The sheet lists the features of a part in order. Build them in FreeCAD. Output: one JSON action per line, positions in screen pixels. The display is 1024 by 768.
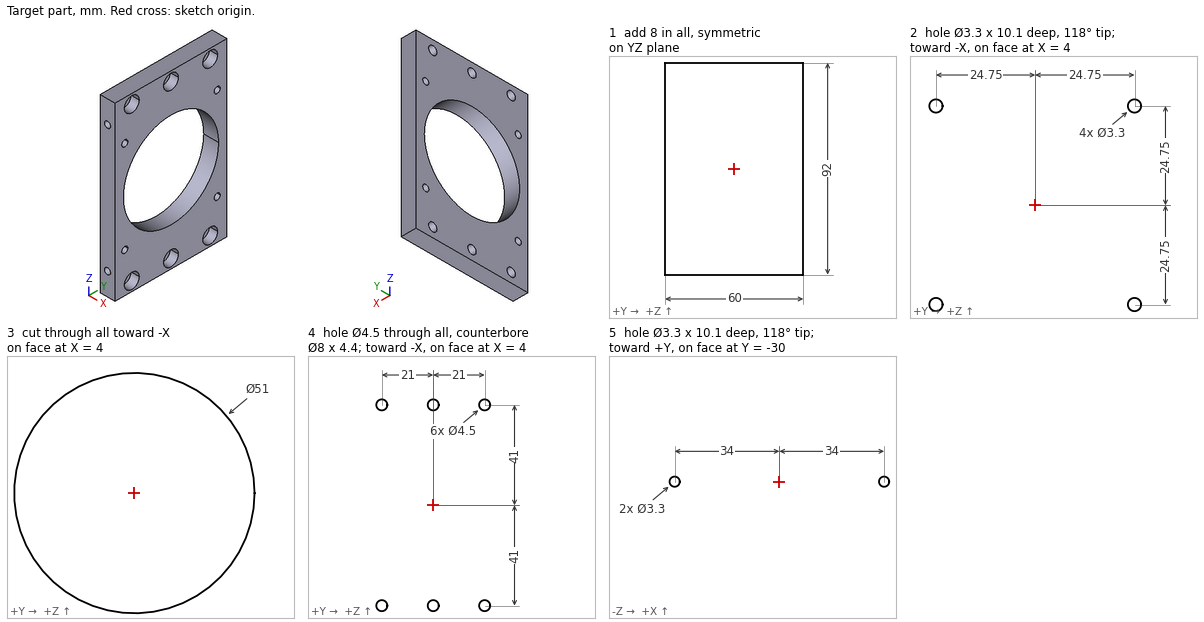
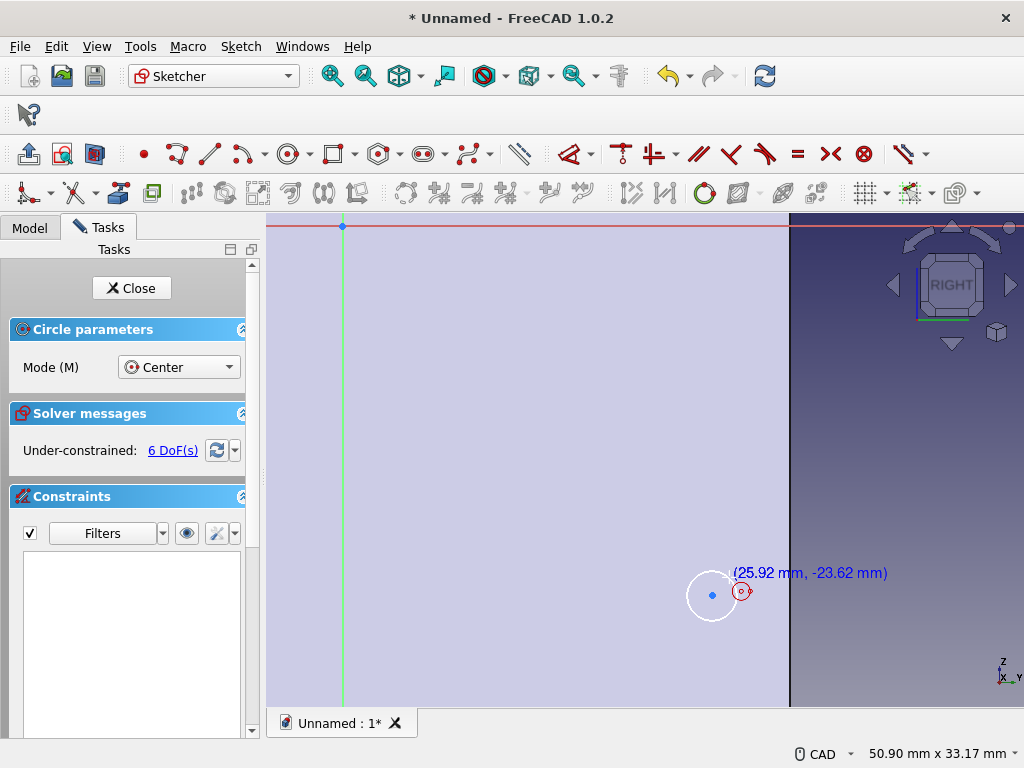
{"action": "scroll", "coordinate": [712, 596], "scroll_direction": "down", "scroll_amount": 5}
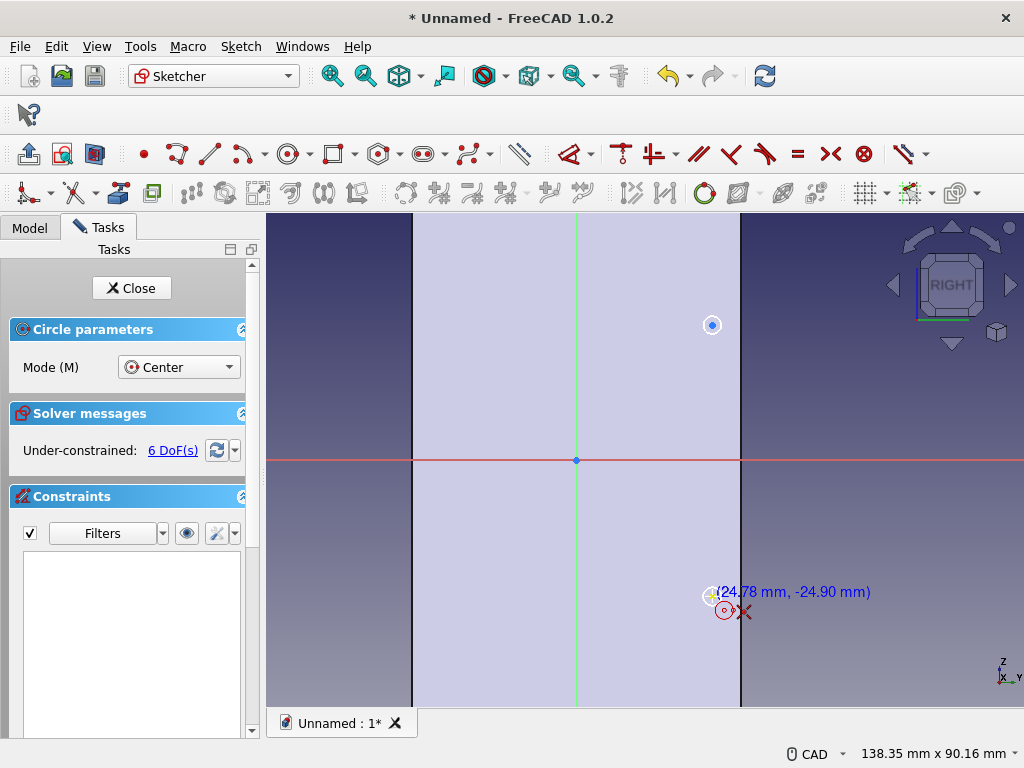
{"action": "scroll", "coordinate": [441, 325], "scroll_direction": "up", "scroll_amount": 5}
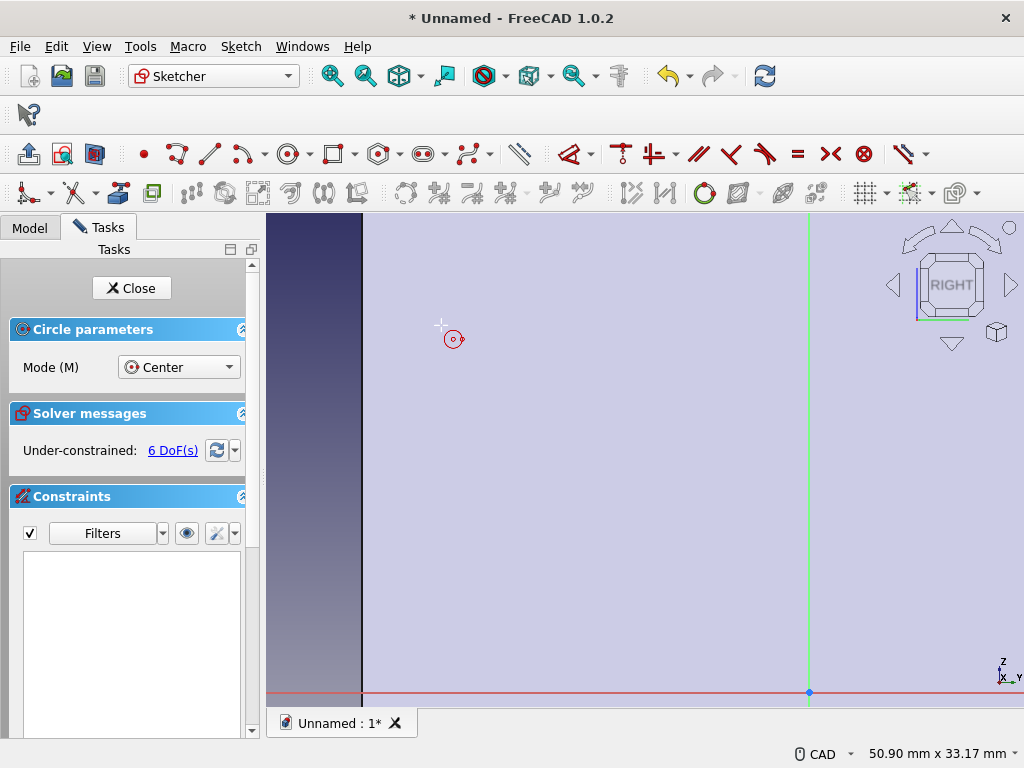
{"action": "left_click", "coordinate": [441, 324]}
{"action": "left_click", "coordinate": [458, 307]}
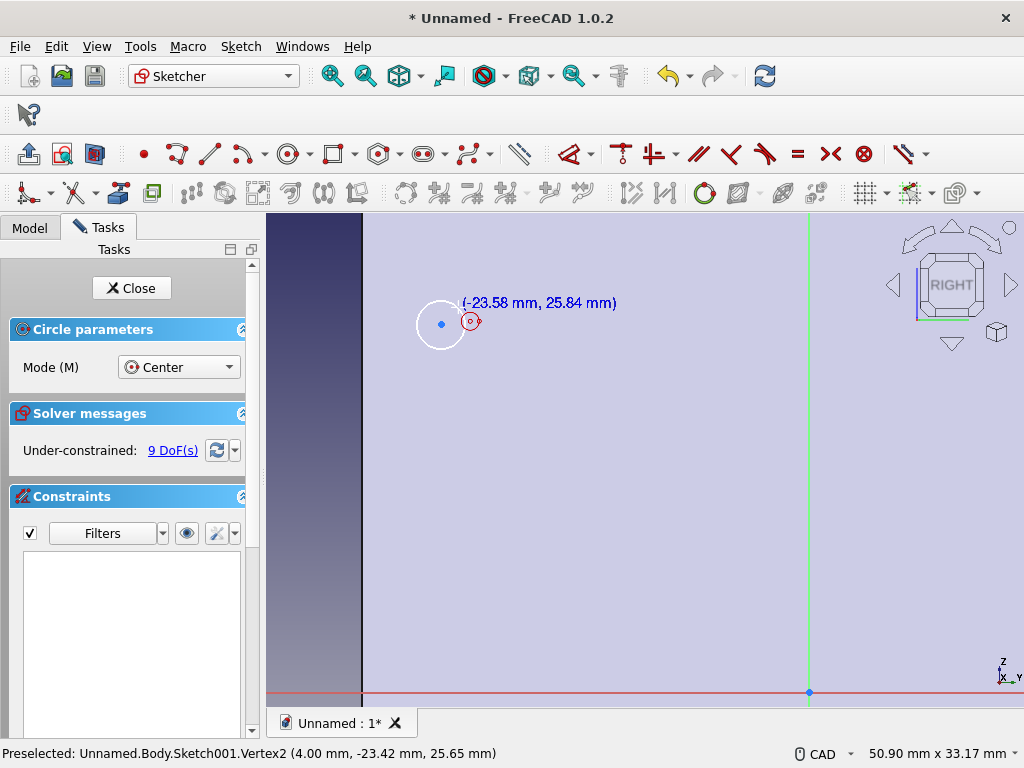
{"action": "scroll", "coordinate": [441, 325], "scroll_direction": "down", "scroll_amount": 5}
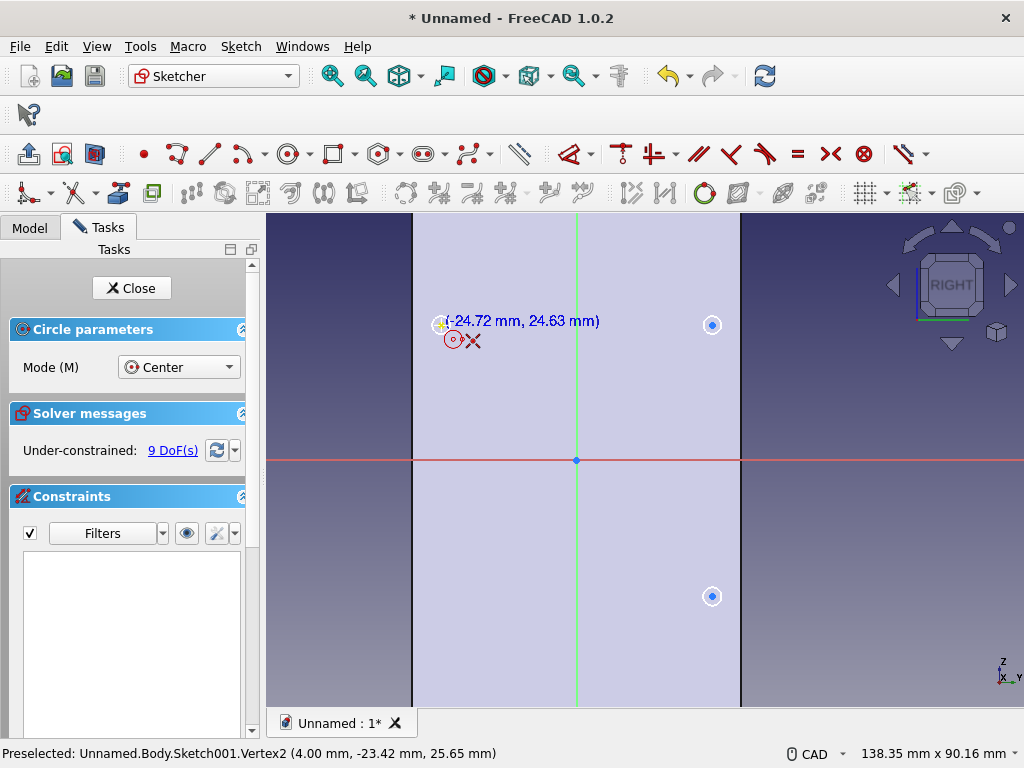
{"action": "scroll", "coordinate": [441, 596], "scroll_direction": "up", "scroll_amount": 5}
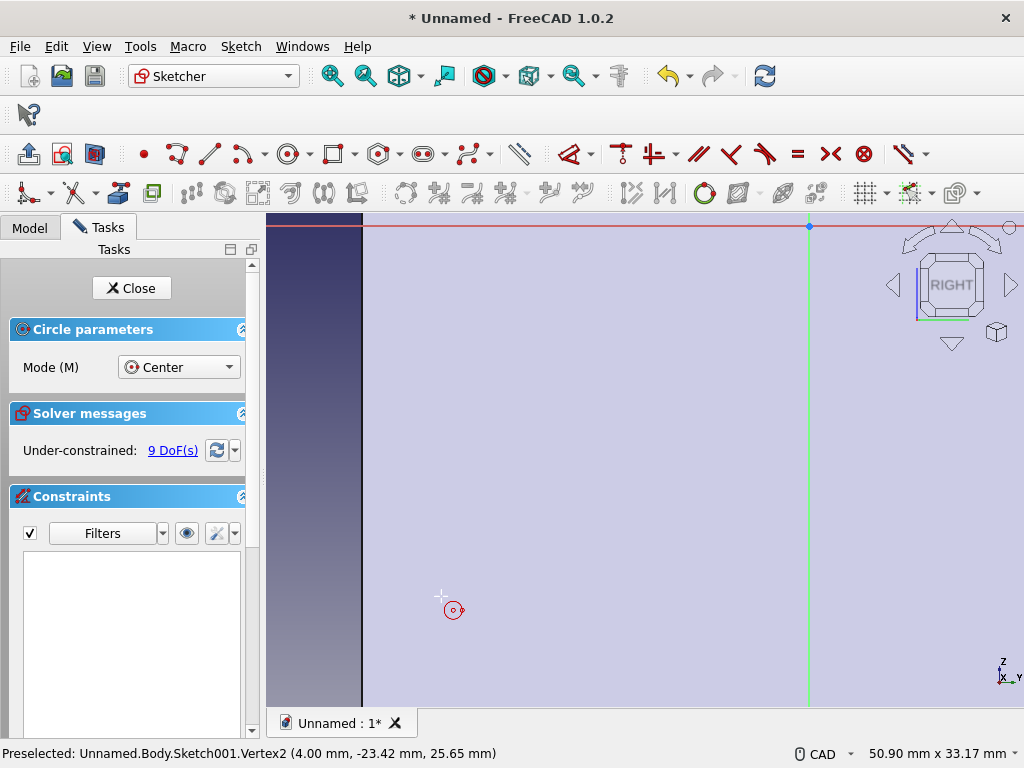
{"action": "left_click", "coordinate": [441, 595]}
{"action": "left_click", "coordinate": [458, 577]}
{"action": "key", "text": "Escape"}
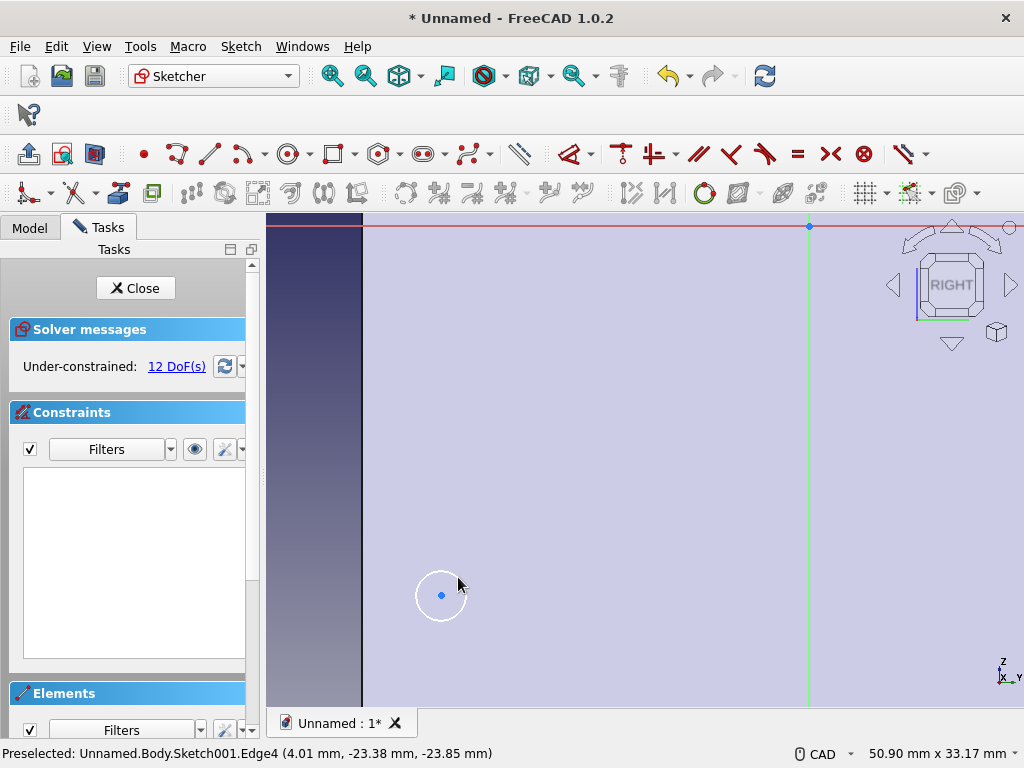
{"action": "scroll", "coordinate": [441, 596], "scroll_direction": "down", "scroll_amount": 5}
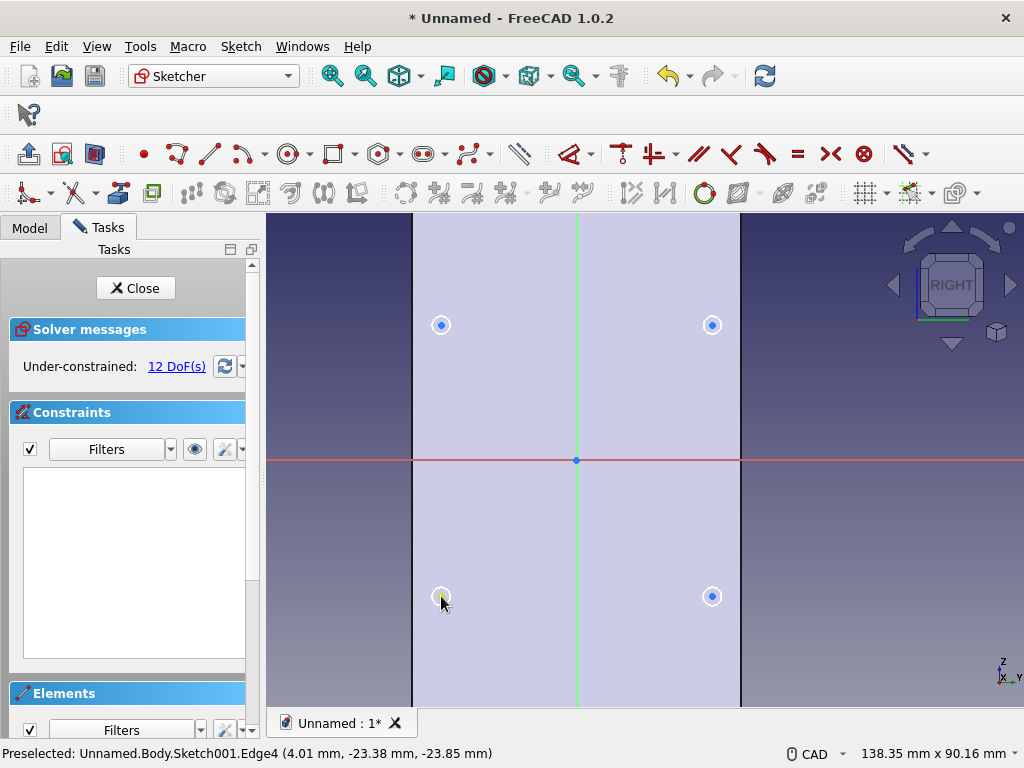
{"action": "scroll", "coordinate": [719, 319], "scroll_direction": "up", "scroll_amount": 3}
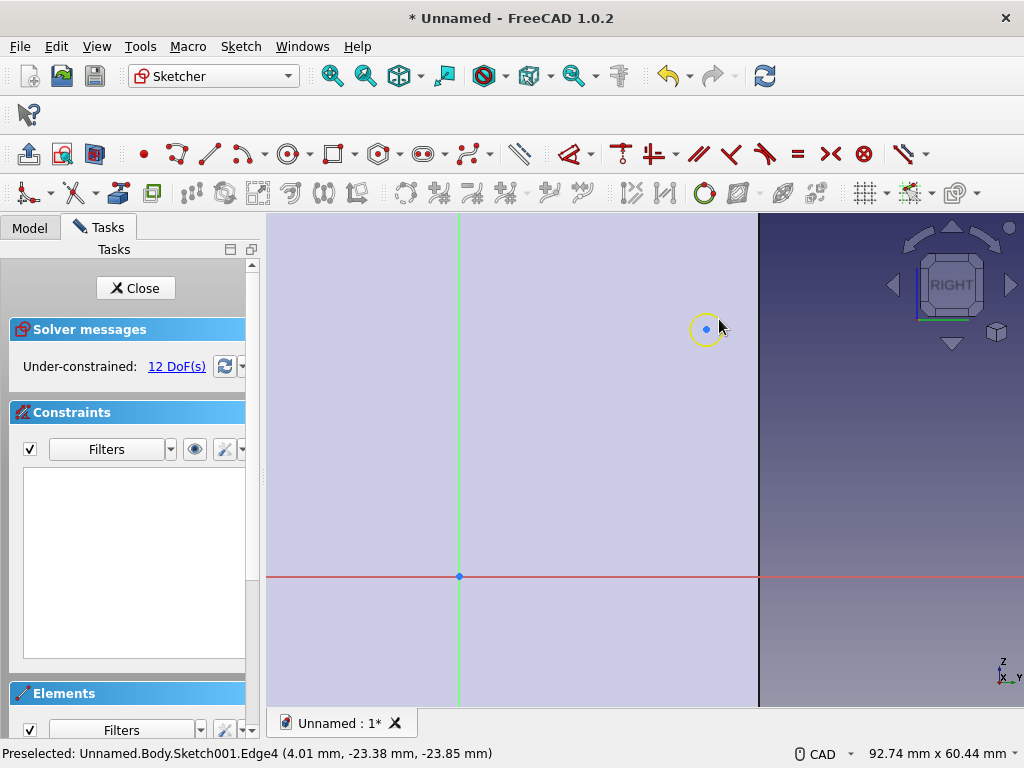
{"action": "left_click", "coordinate": [718, 319]}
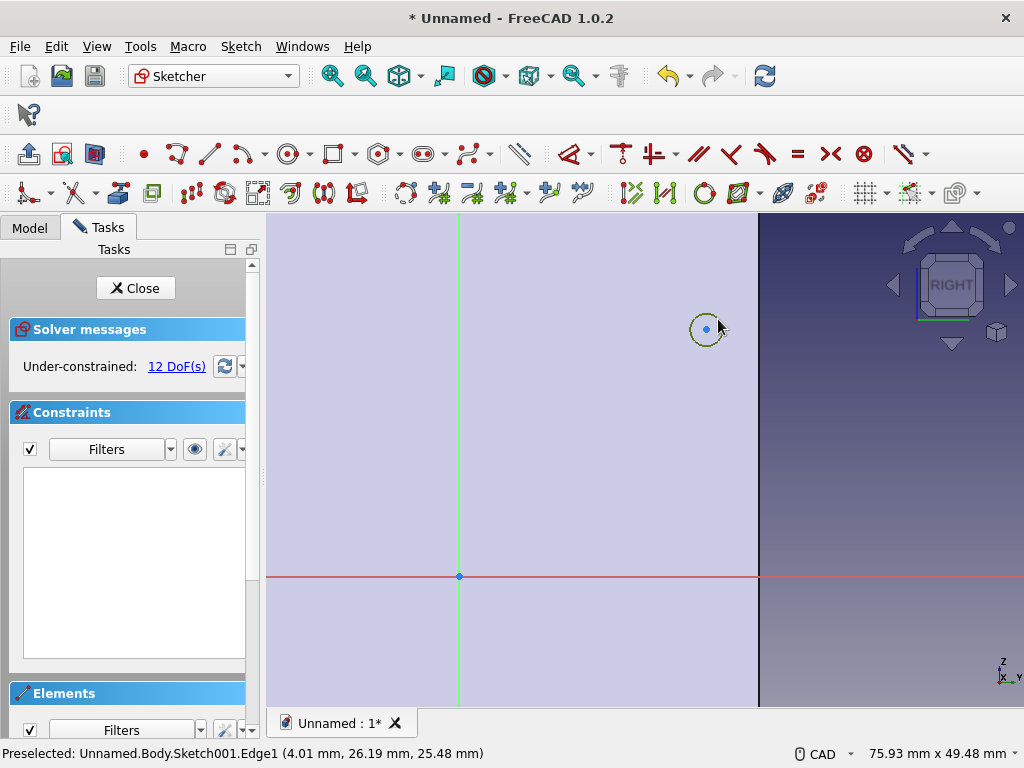
{"action": "scroll", "coordinate": [719, 318], "scroll_direction": "down", "scroll_amount": 3}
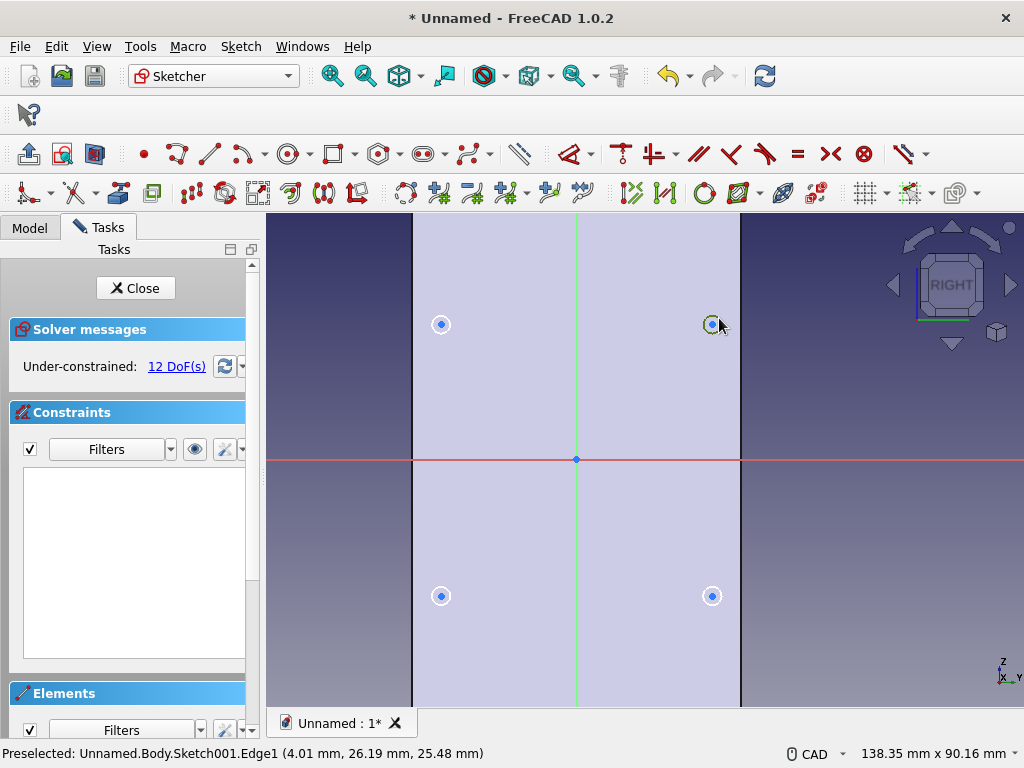
{"action": "scroll", "coordinate": [719, 590], "scroll_direction": "up", "scroll_amount": 3}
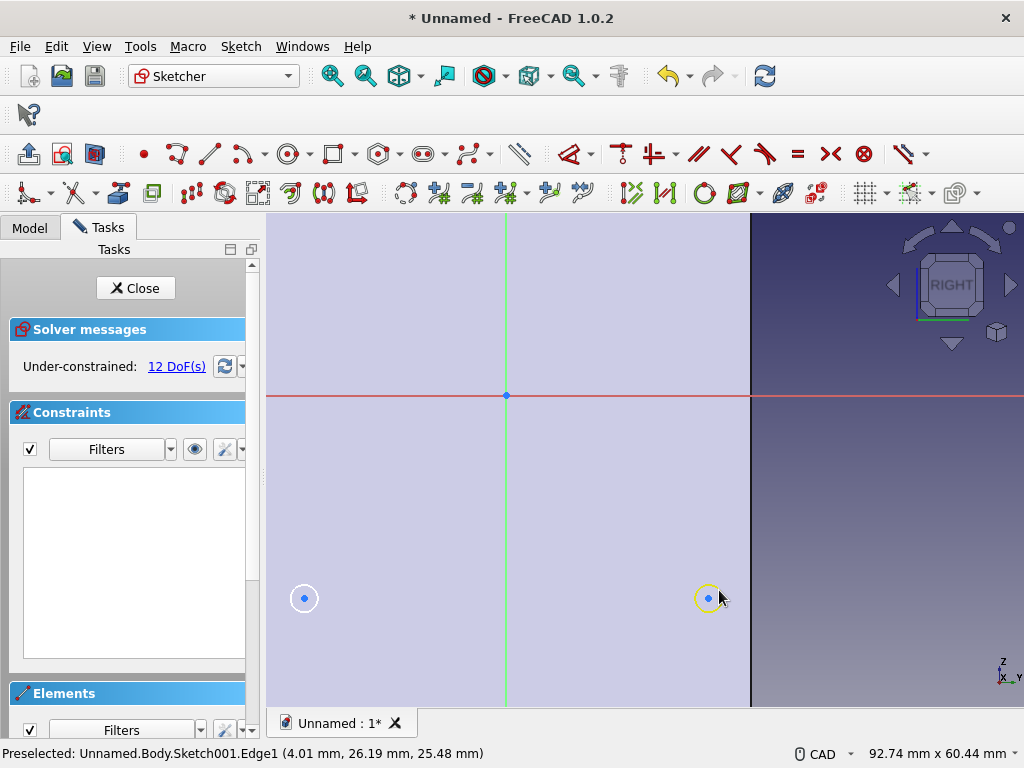
{"action": "left_click", "coordinate": [718, 589]}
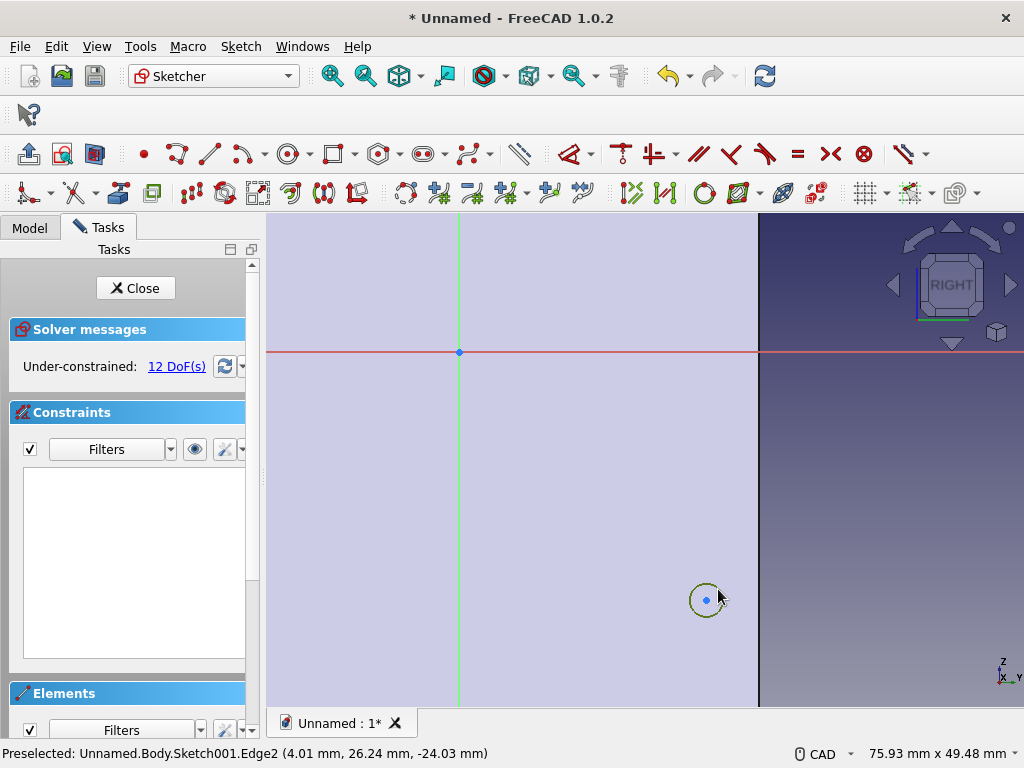
{"action": "scroll", "coordinate": [719, 591], "scroll_direction": "down", "scroll_amount": 3}